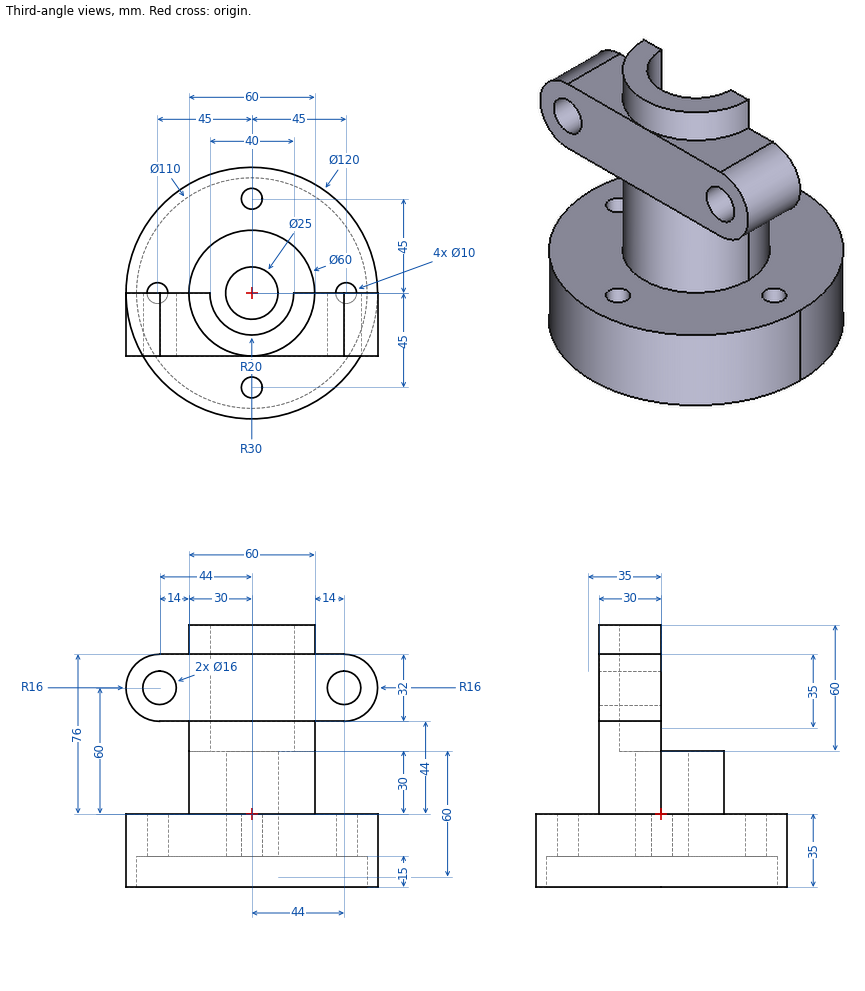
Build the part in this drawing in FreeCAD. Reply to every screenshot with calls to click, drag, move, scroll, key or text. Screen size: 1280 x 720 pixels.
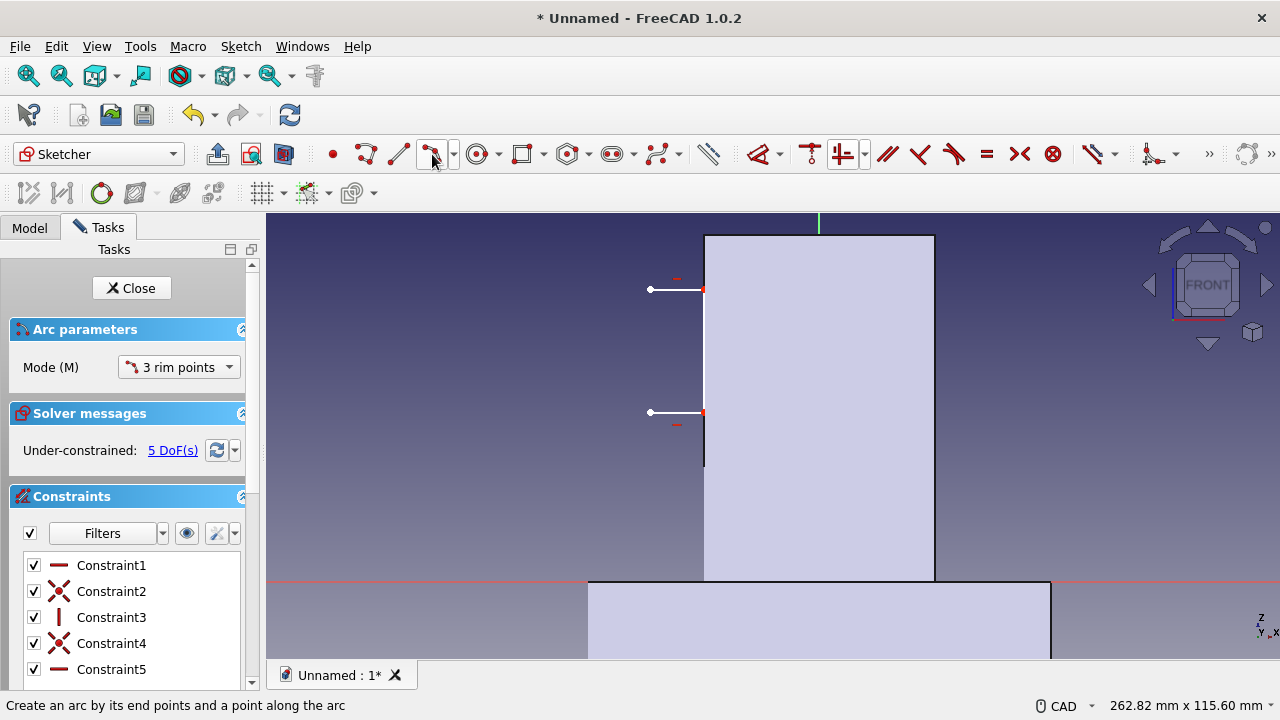
click(650, 413)
click(650, 290)
click(588, 351)
key(Escape)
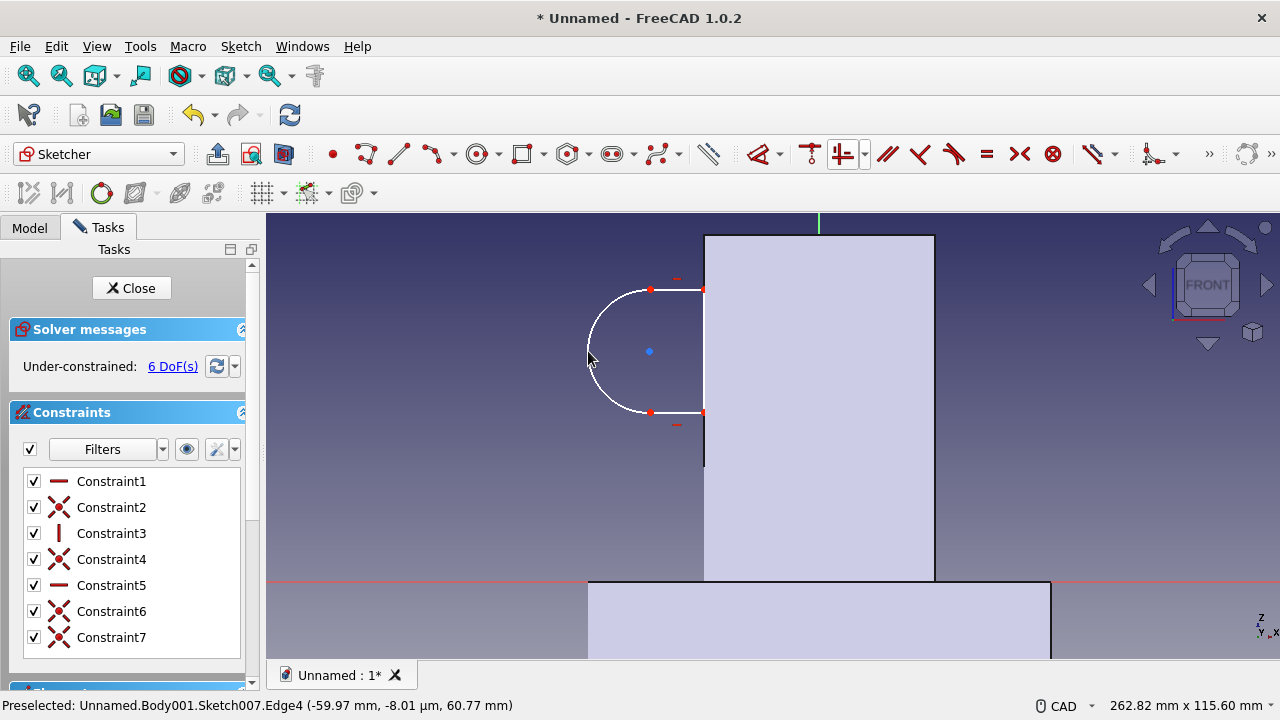
click(666, 290)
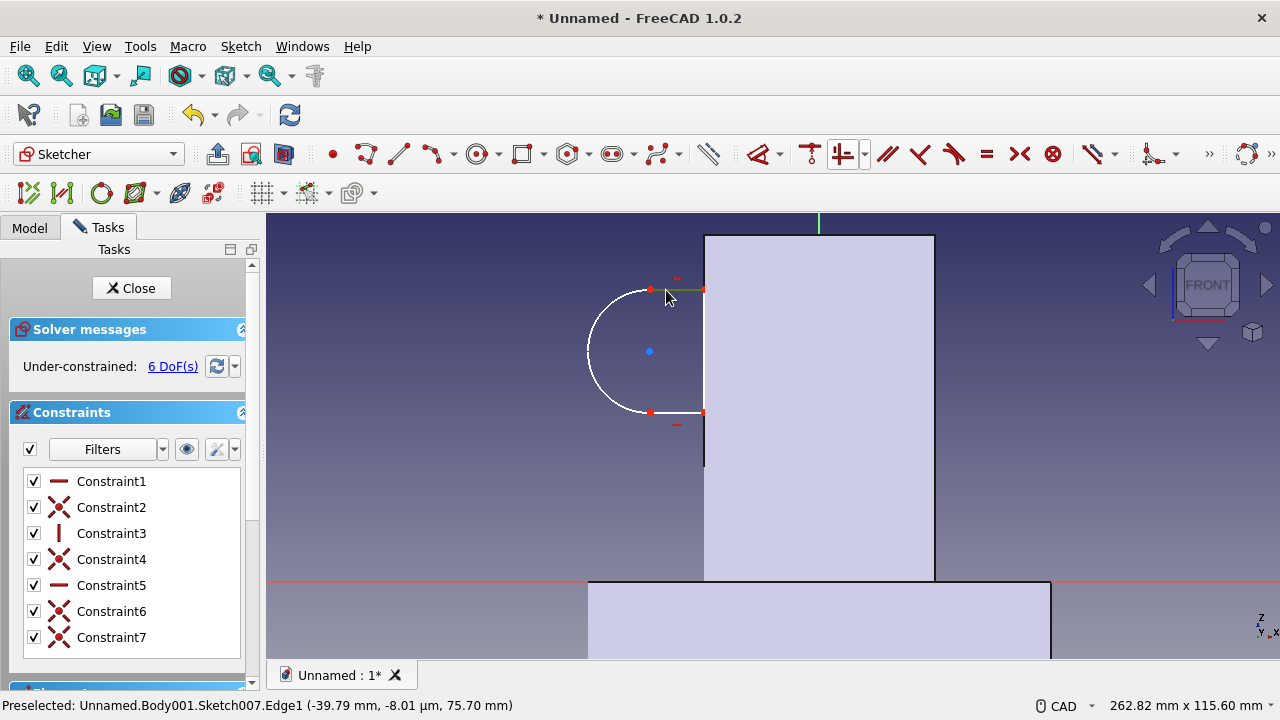
click(600, 315)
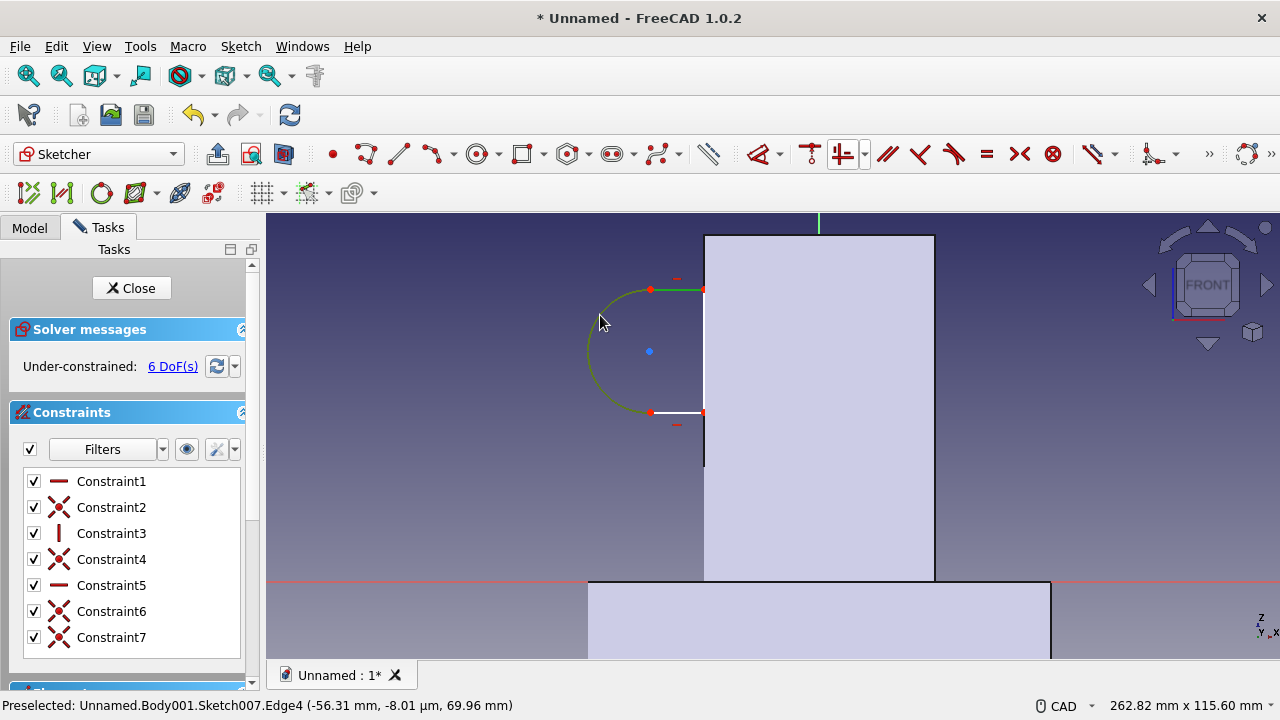
click(954, 154)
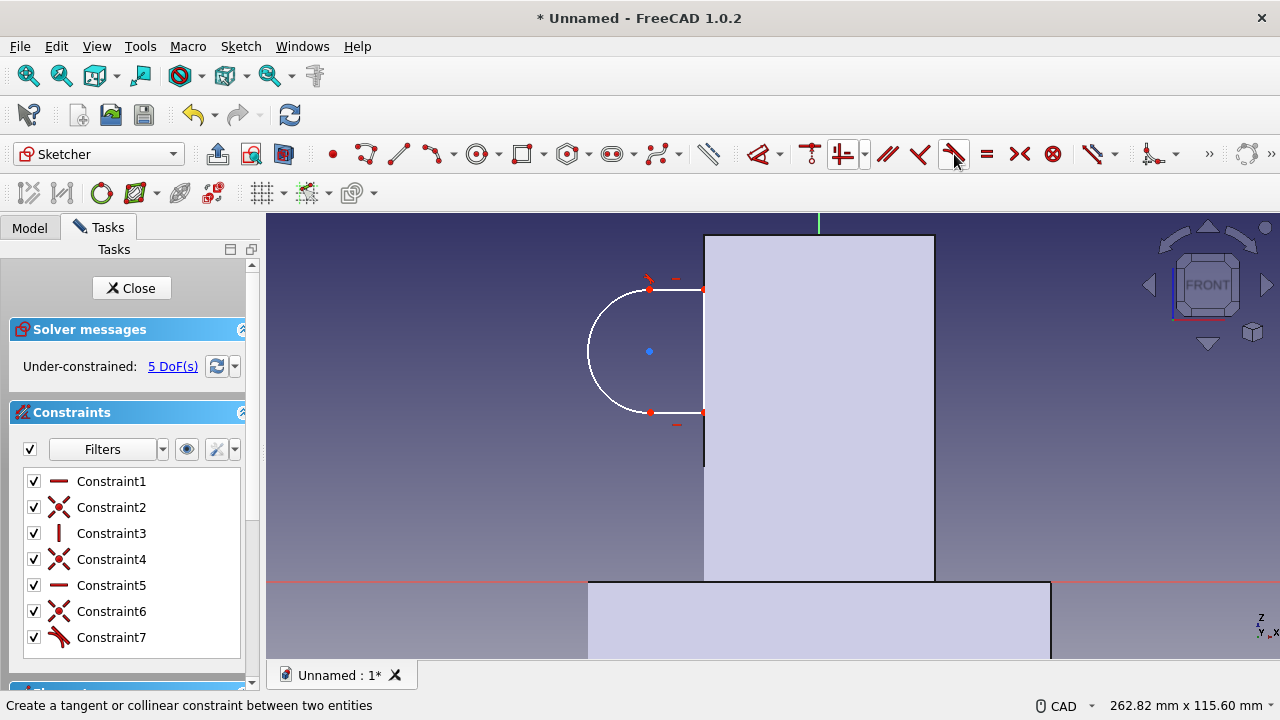
click(688, 413)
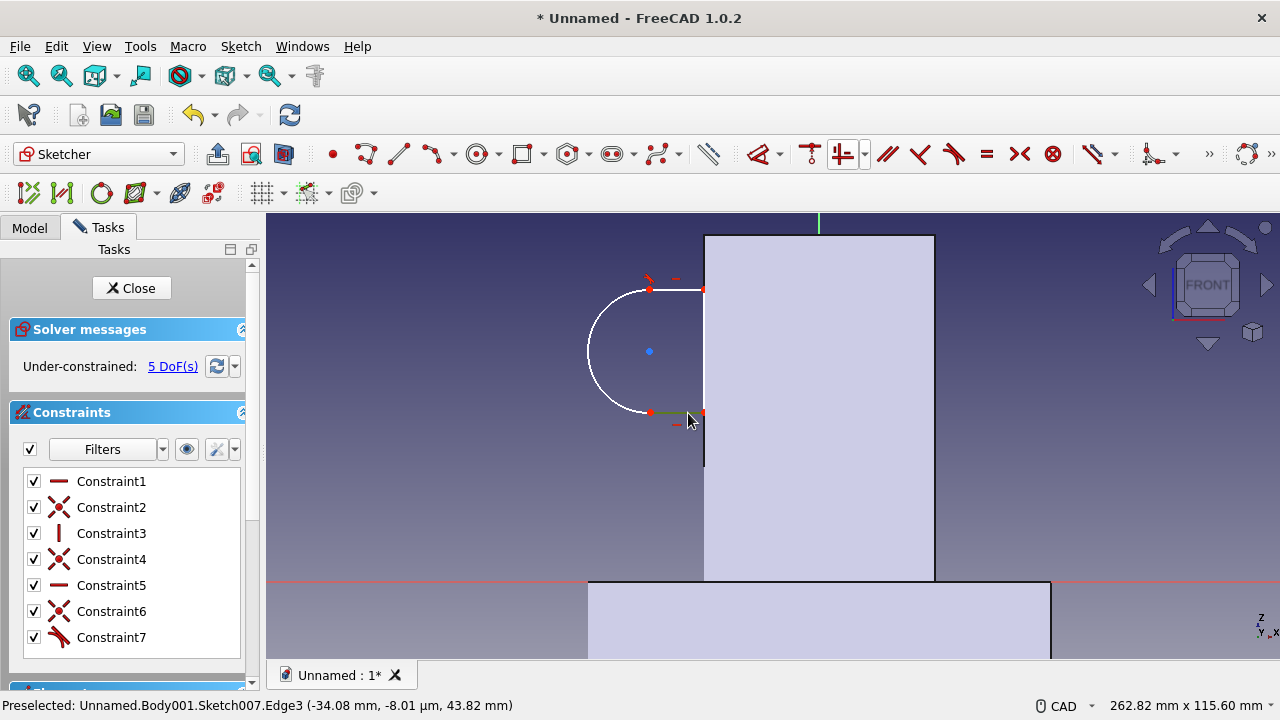
click(600, 315)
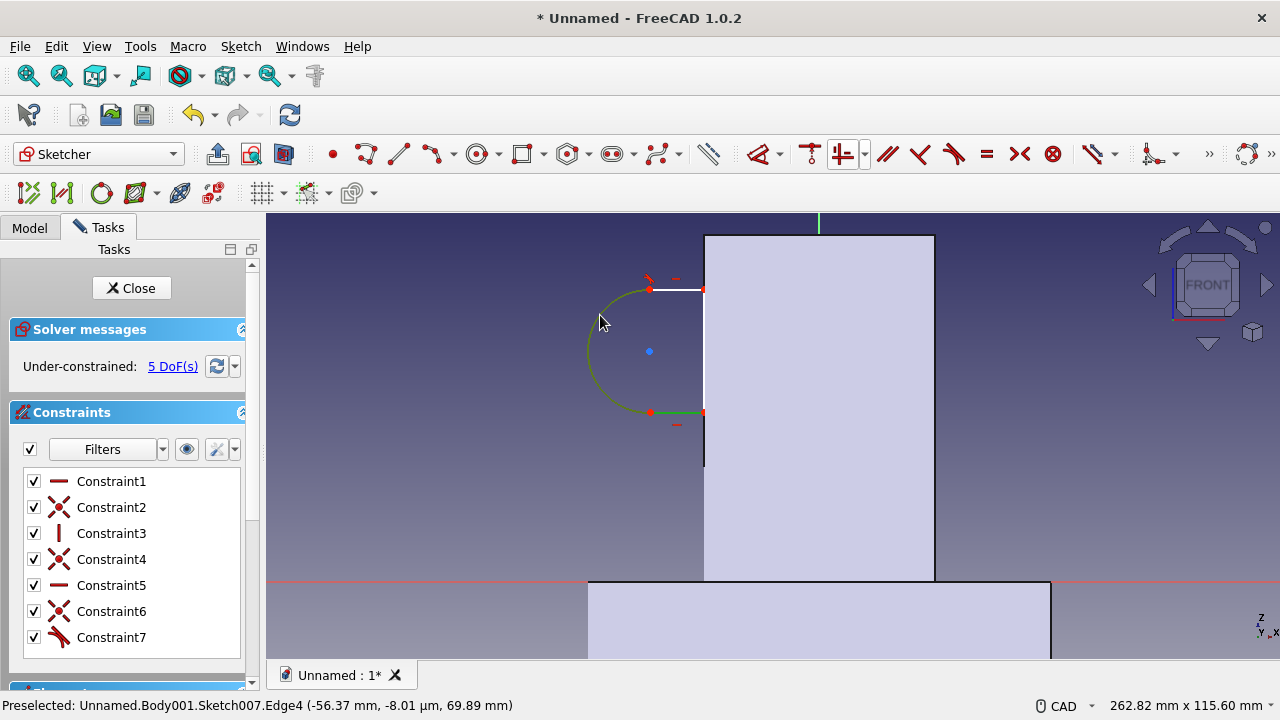
click(954, 154)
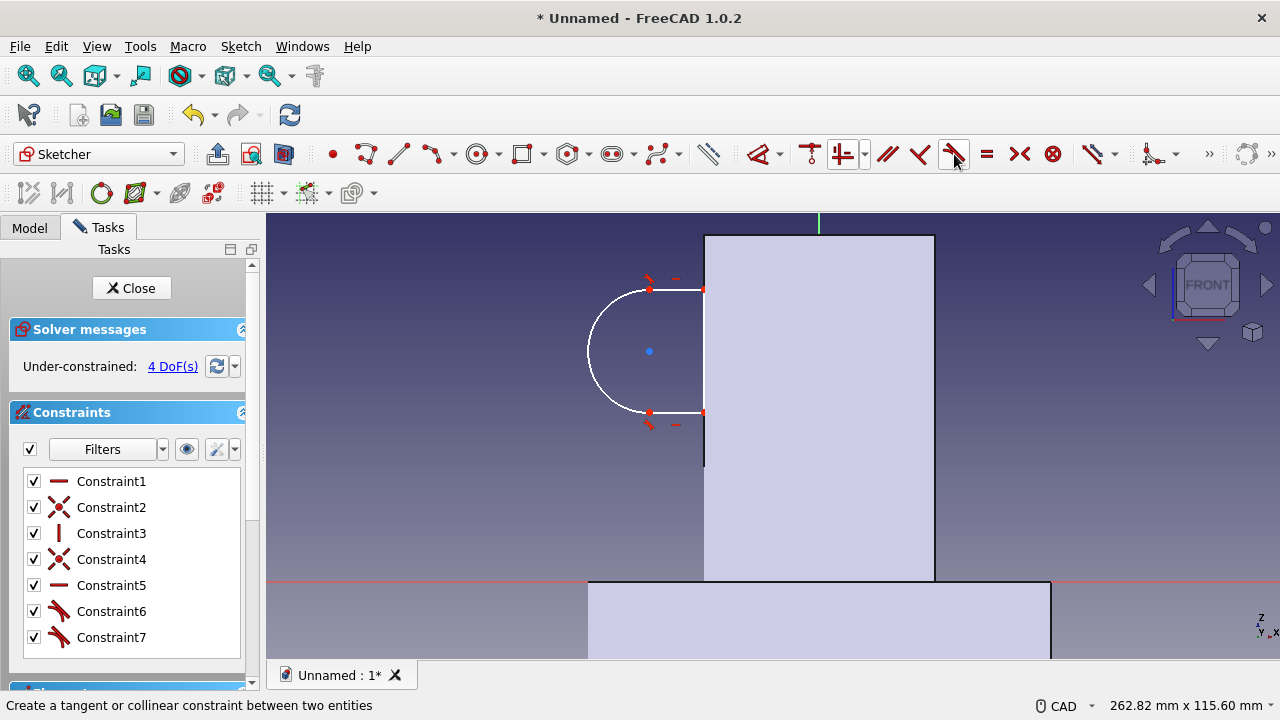
click(758, 154)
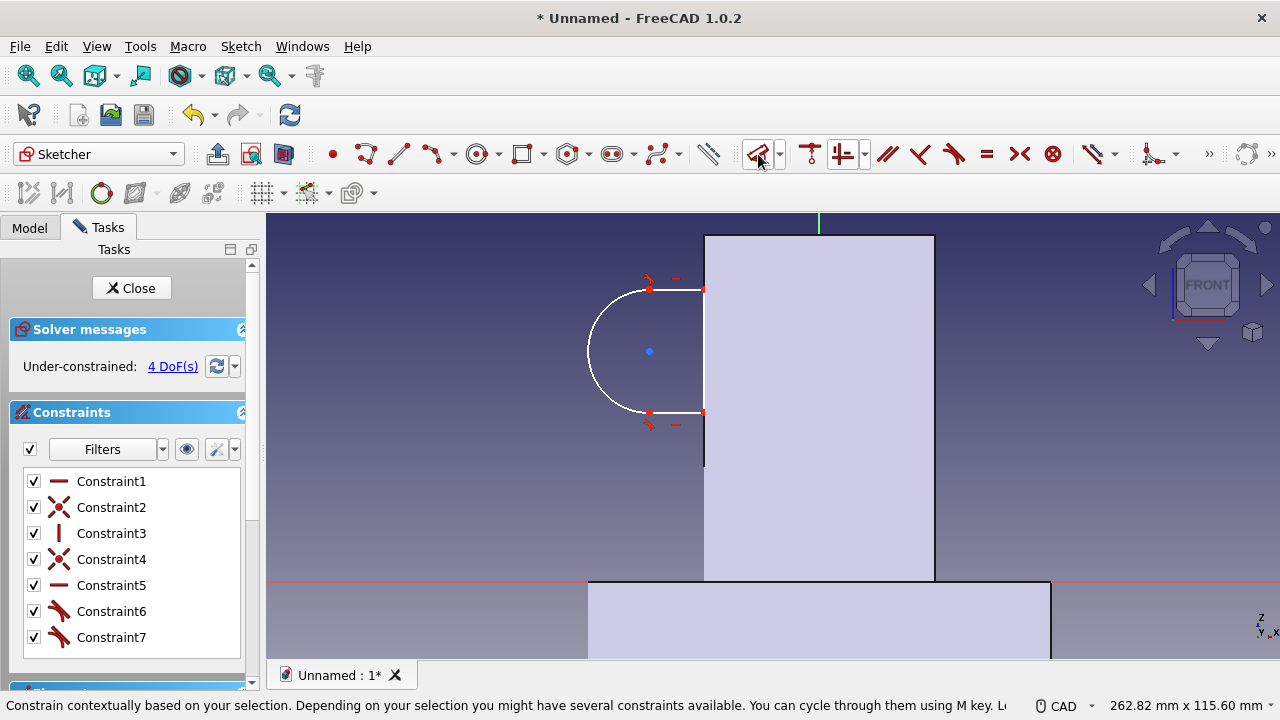
click(600, 315)
click(574, 296)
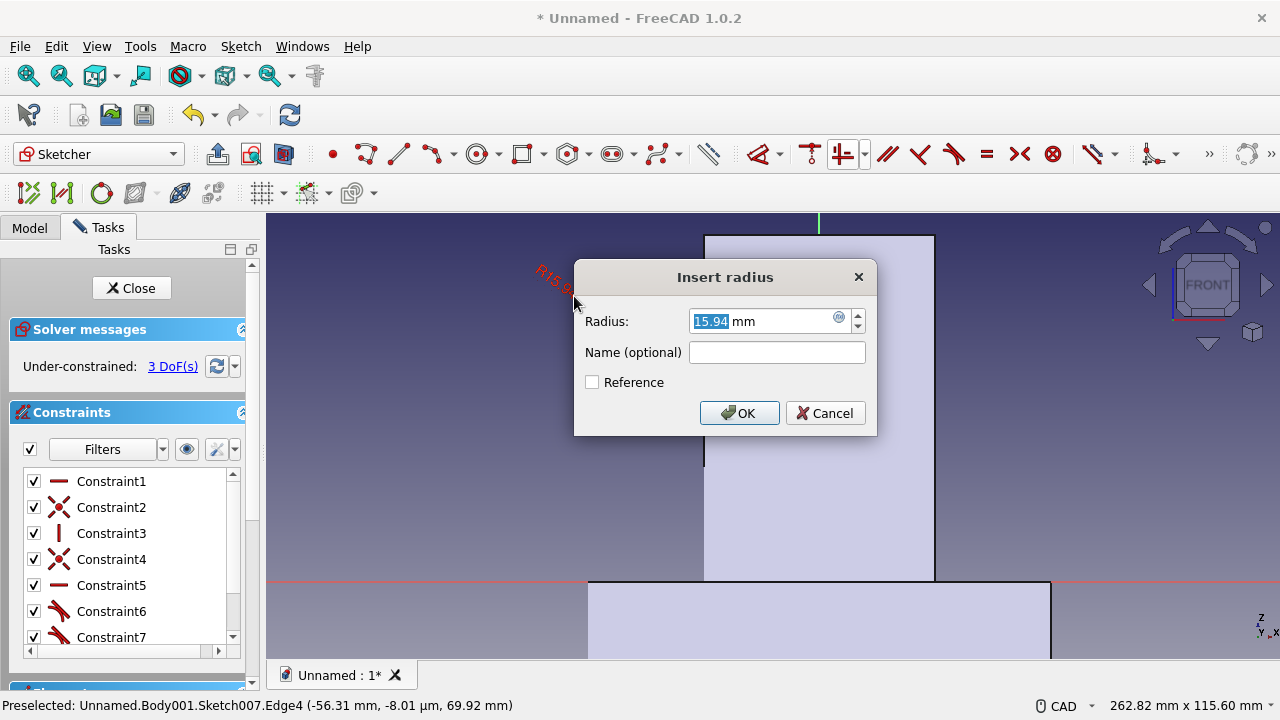
text(16)
key(Return)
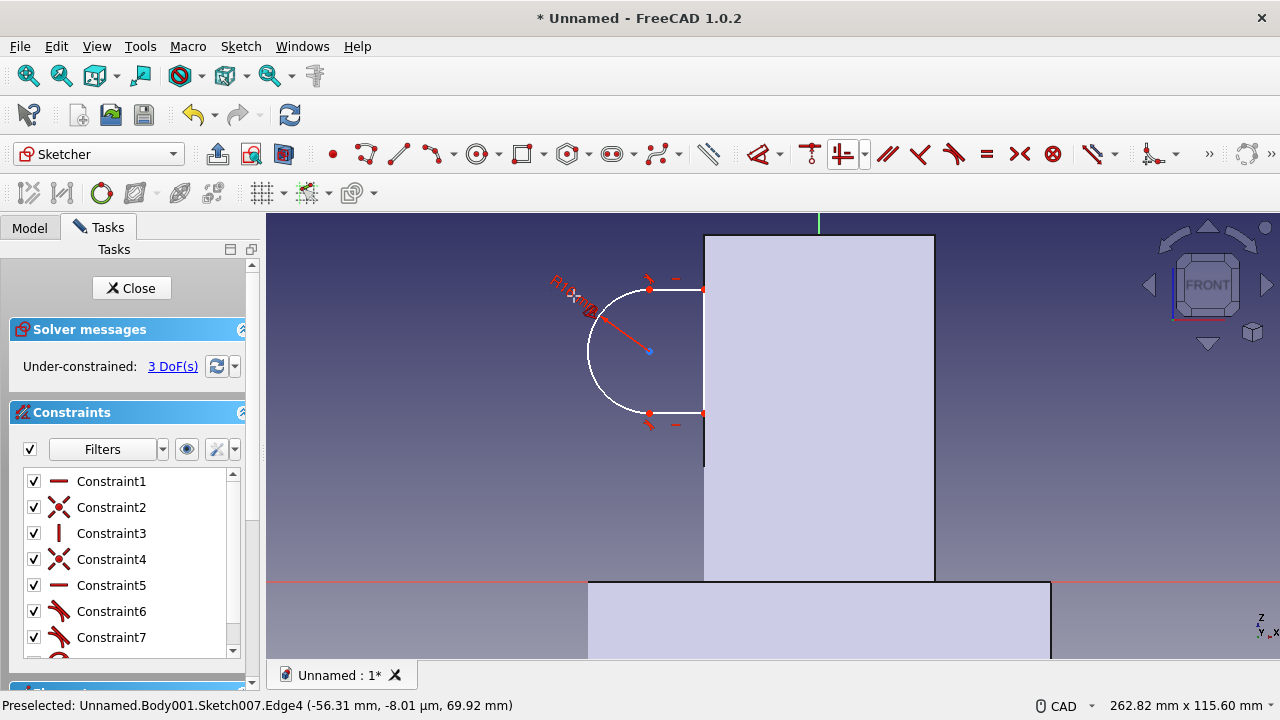
click(666, 290)
click(677, 256)